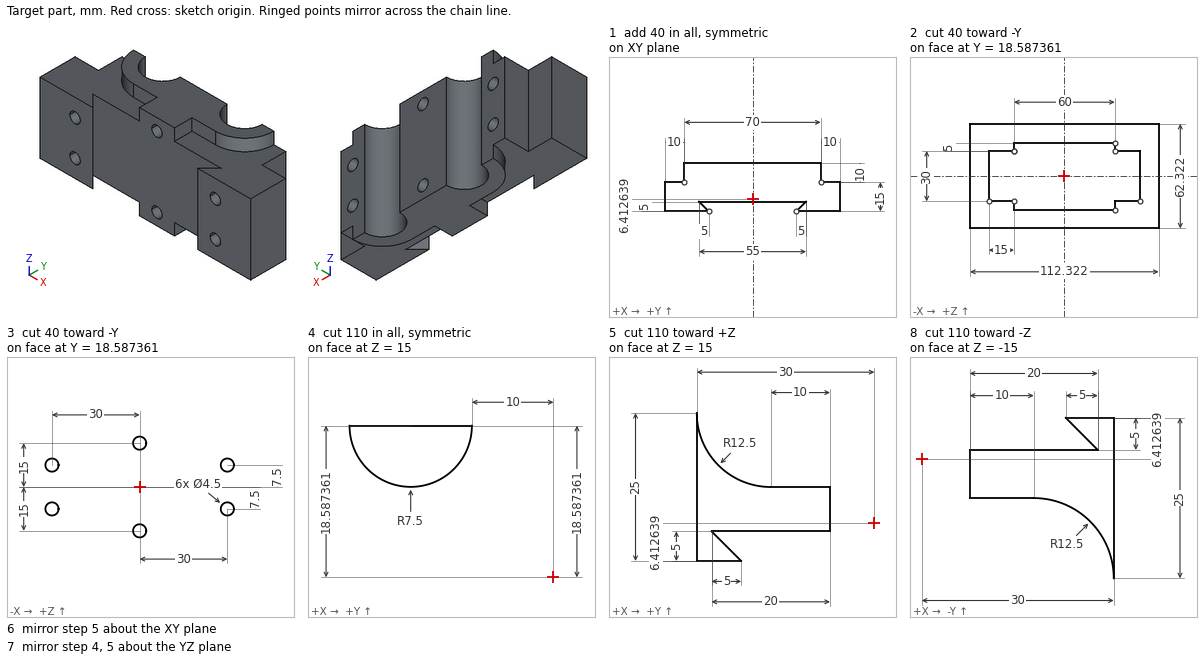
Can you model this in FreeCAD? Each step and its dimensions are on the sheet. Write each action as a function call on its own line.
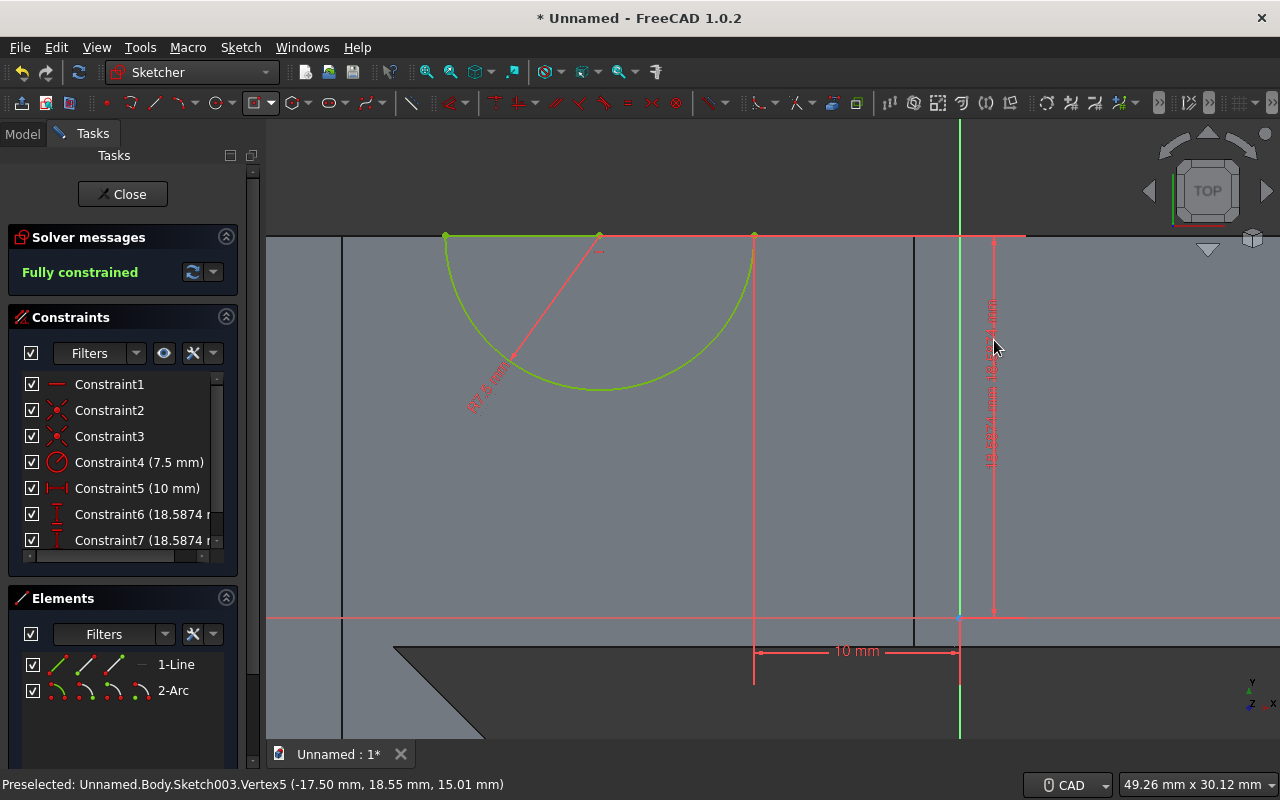
click(123, 194)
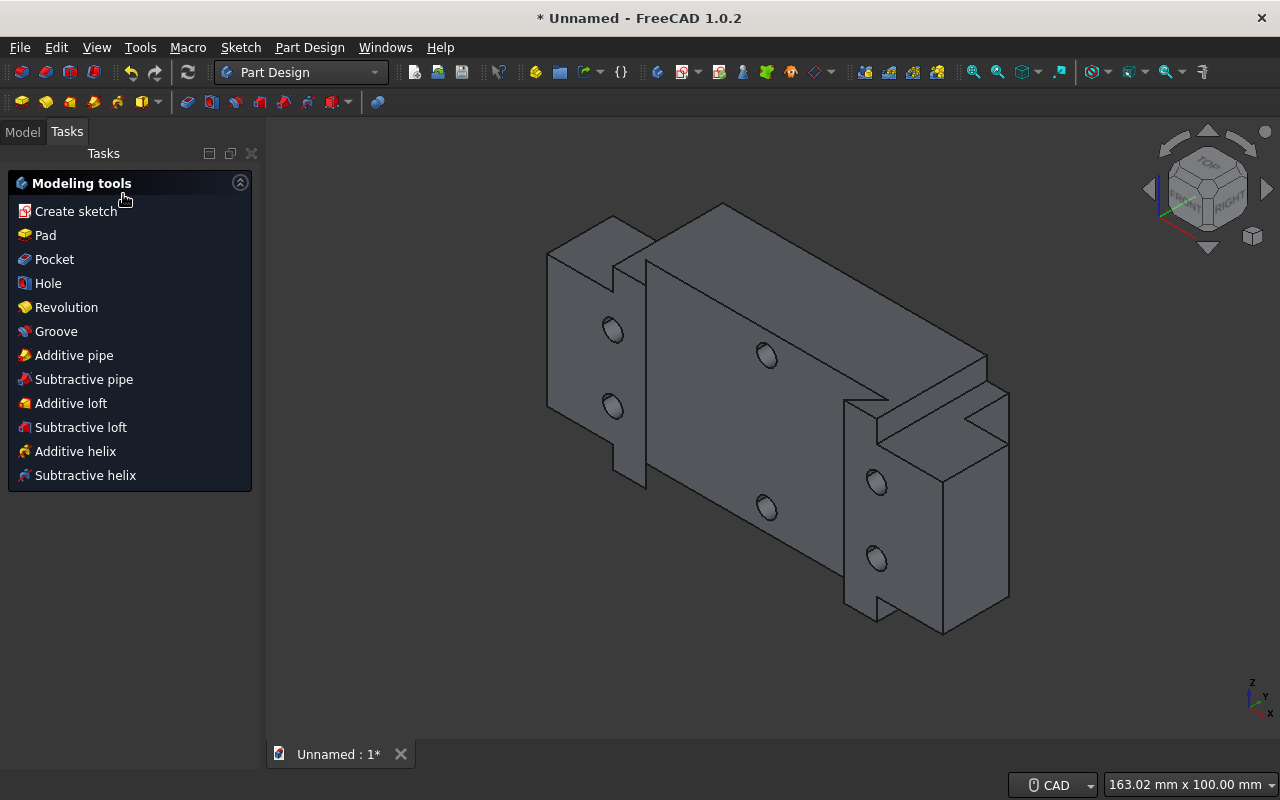
click(188, 102)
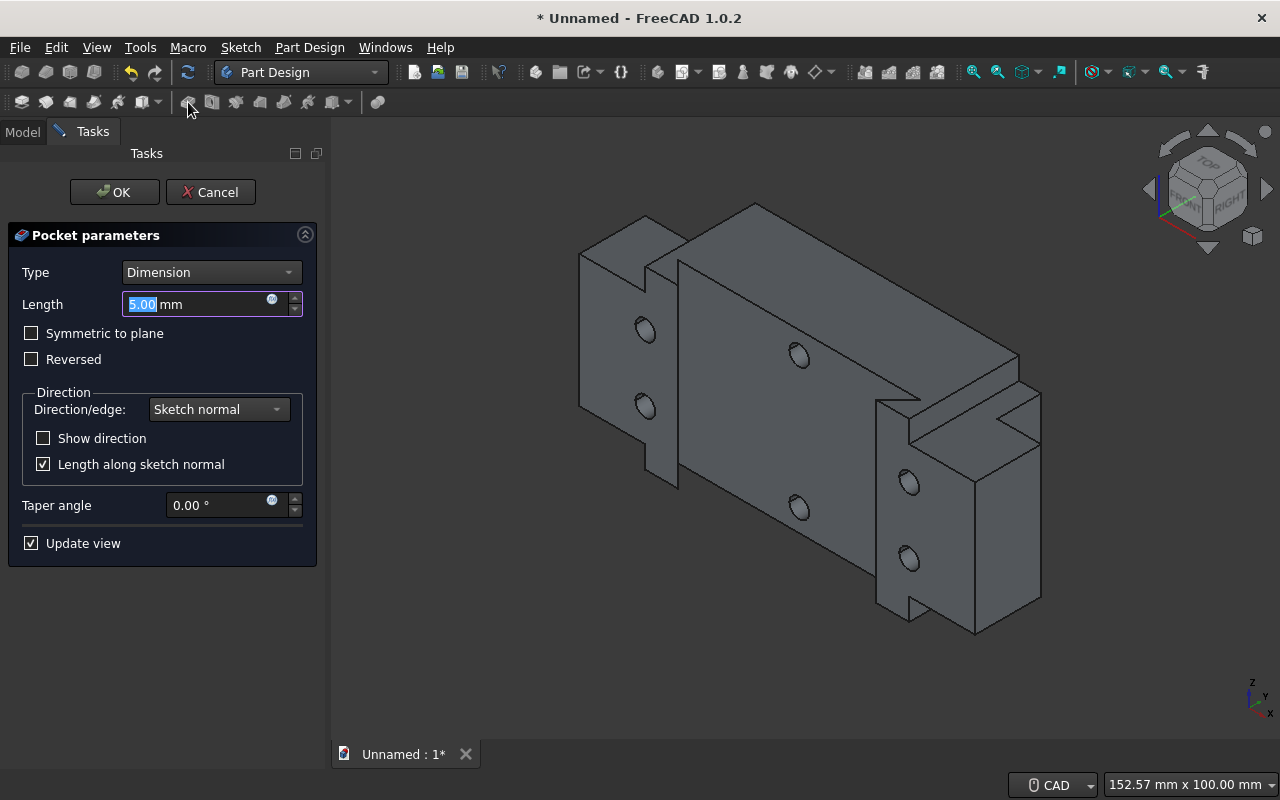
text(110)
key(Tab)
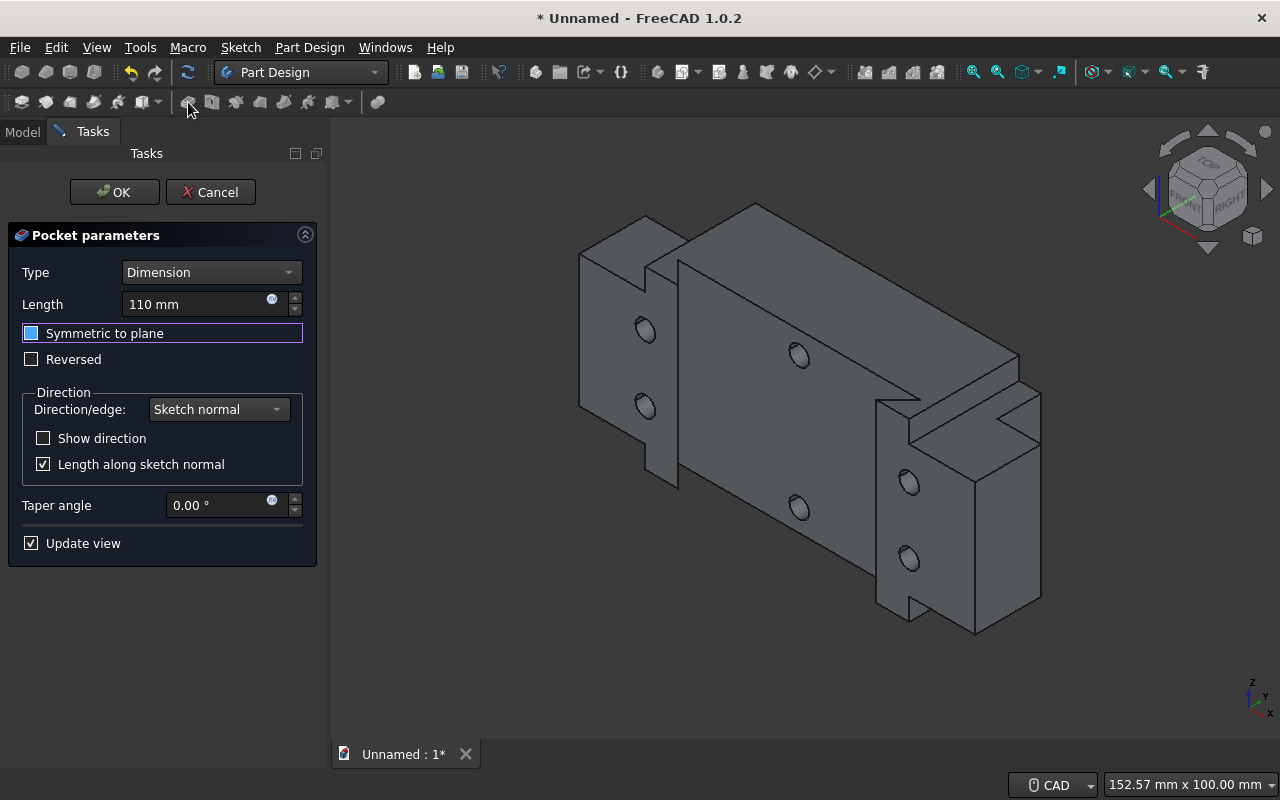
click(30, 333)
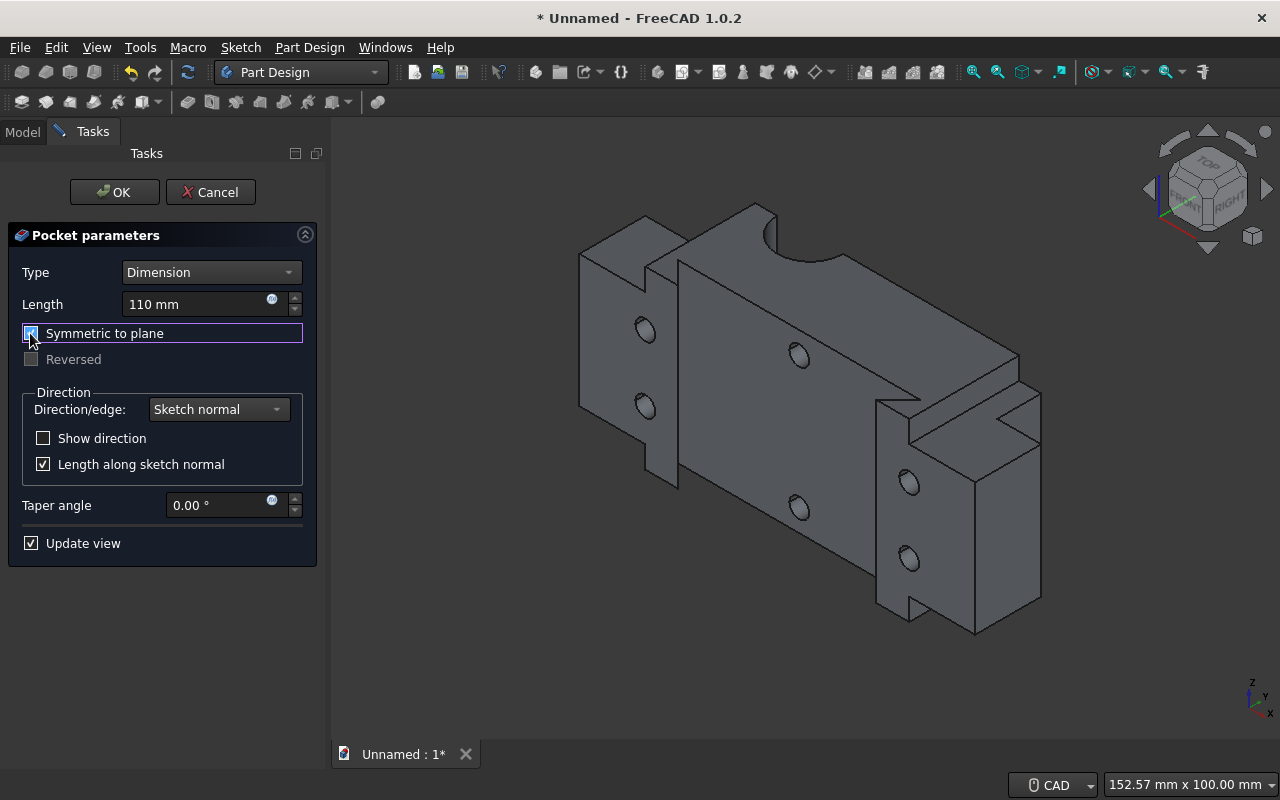
click(115, 192)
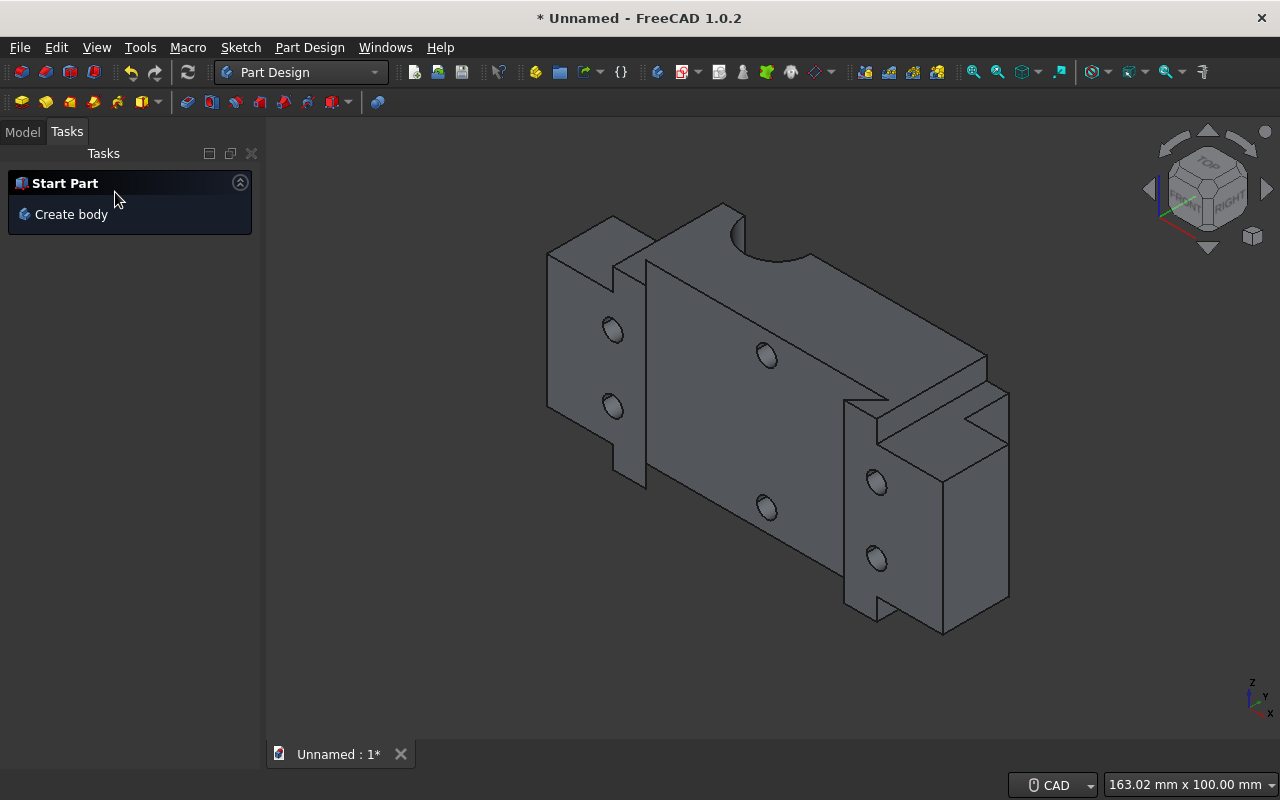
click(949, 440)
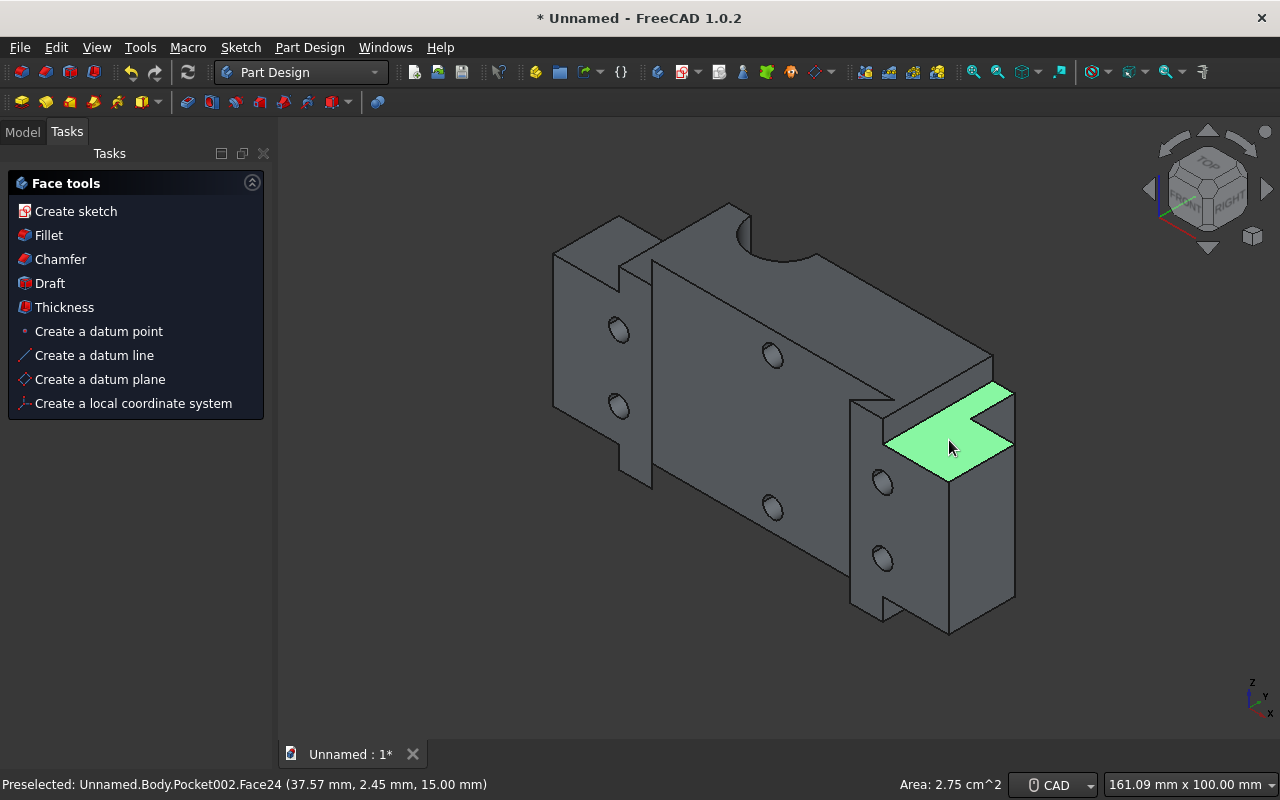
click(682, 72)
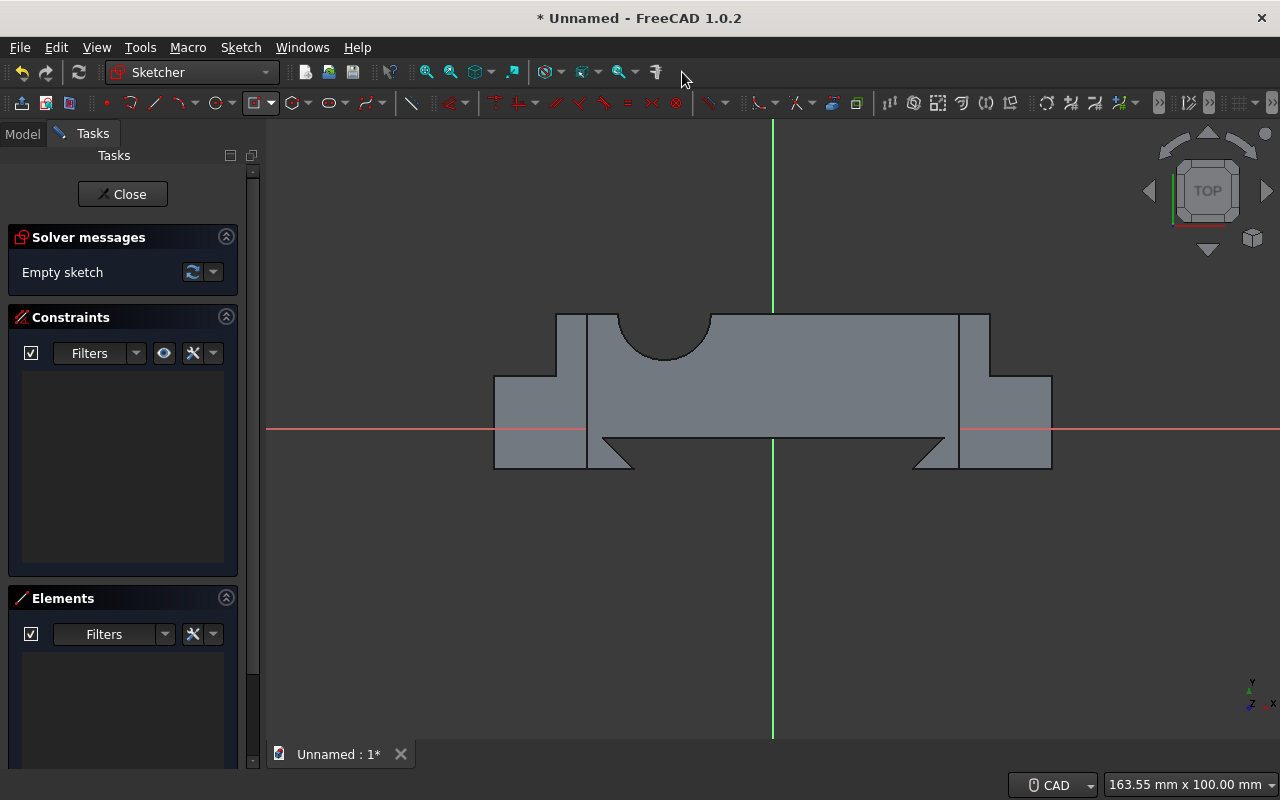
scroll(666, 369, up, 5)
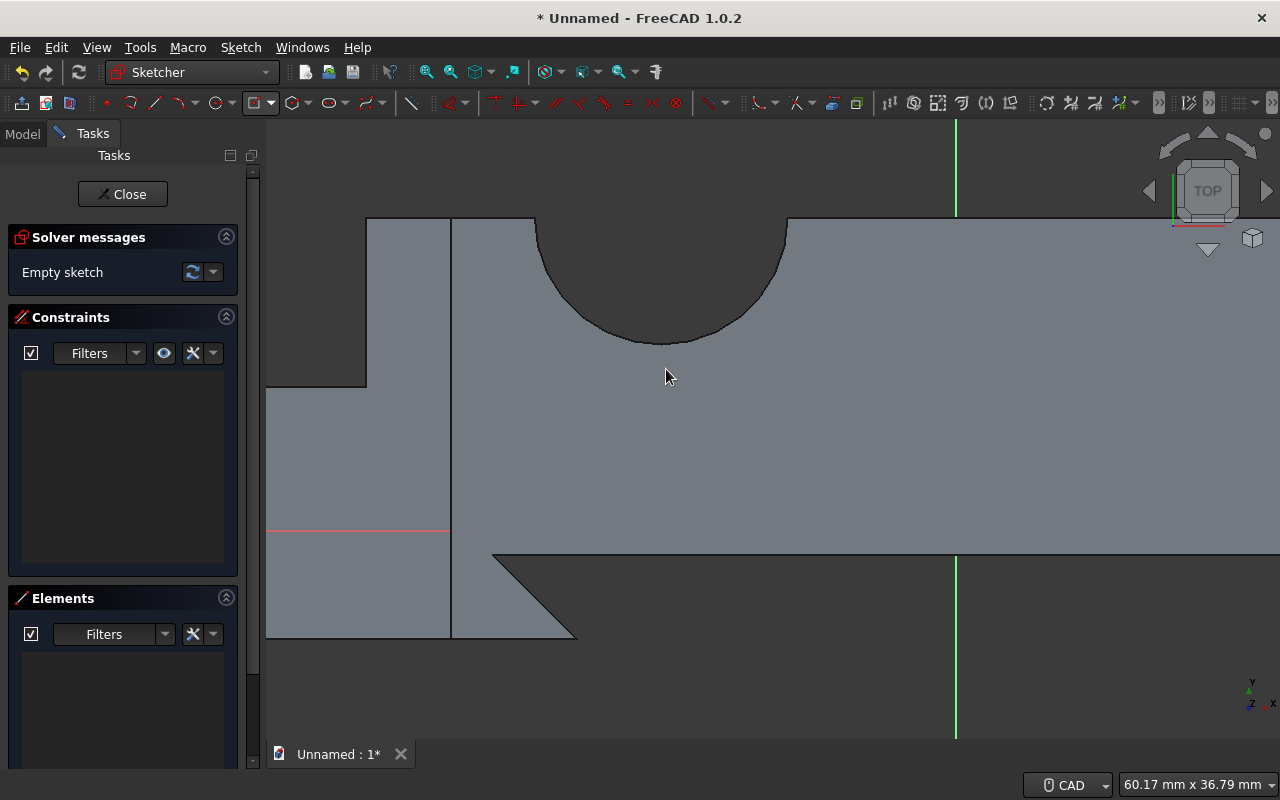
key(g)
key(m)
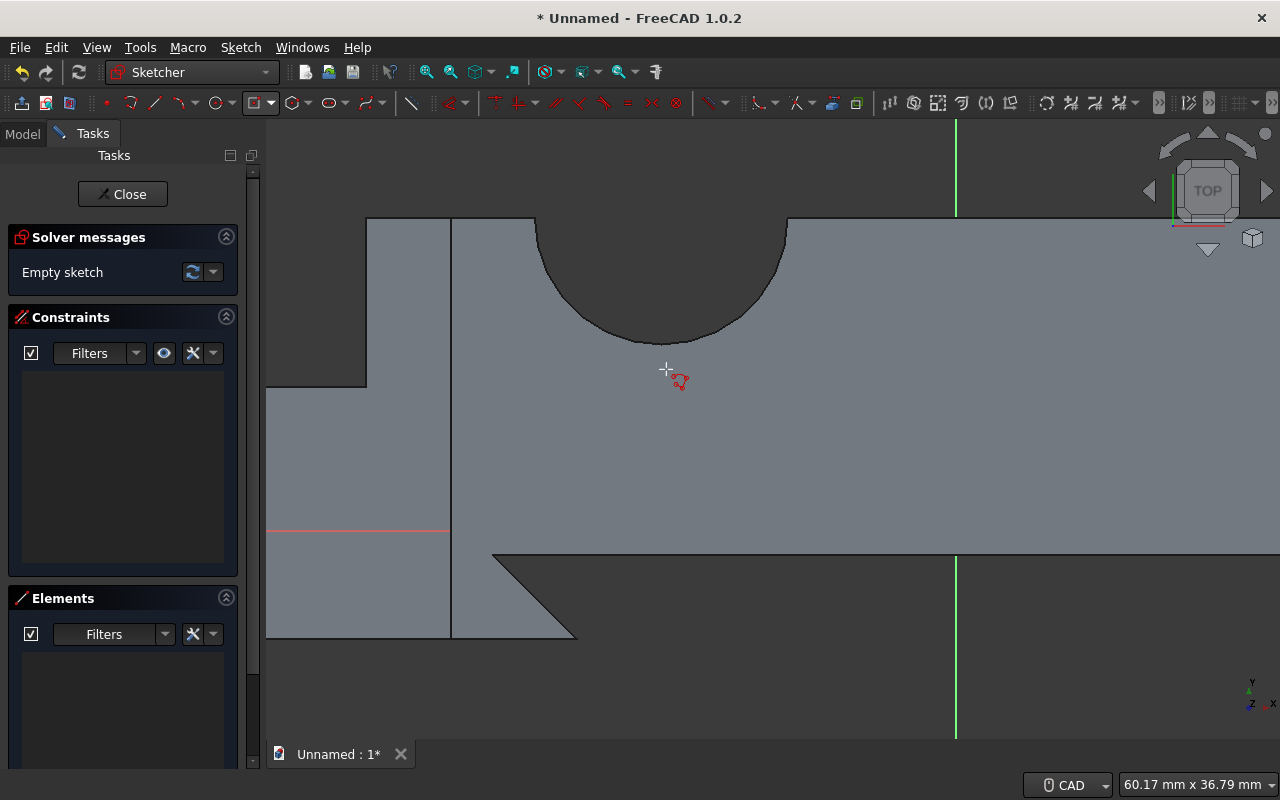
click(451, 218)
click(451, 639)
click(577, 639)
click(493, 555)
click(830, 555)
click(830, 429)
click(661, 429)
right_click(661, 429)